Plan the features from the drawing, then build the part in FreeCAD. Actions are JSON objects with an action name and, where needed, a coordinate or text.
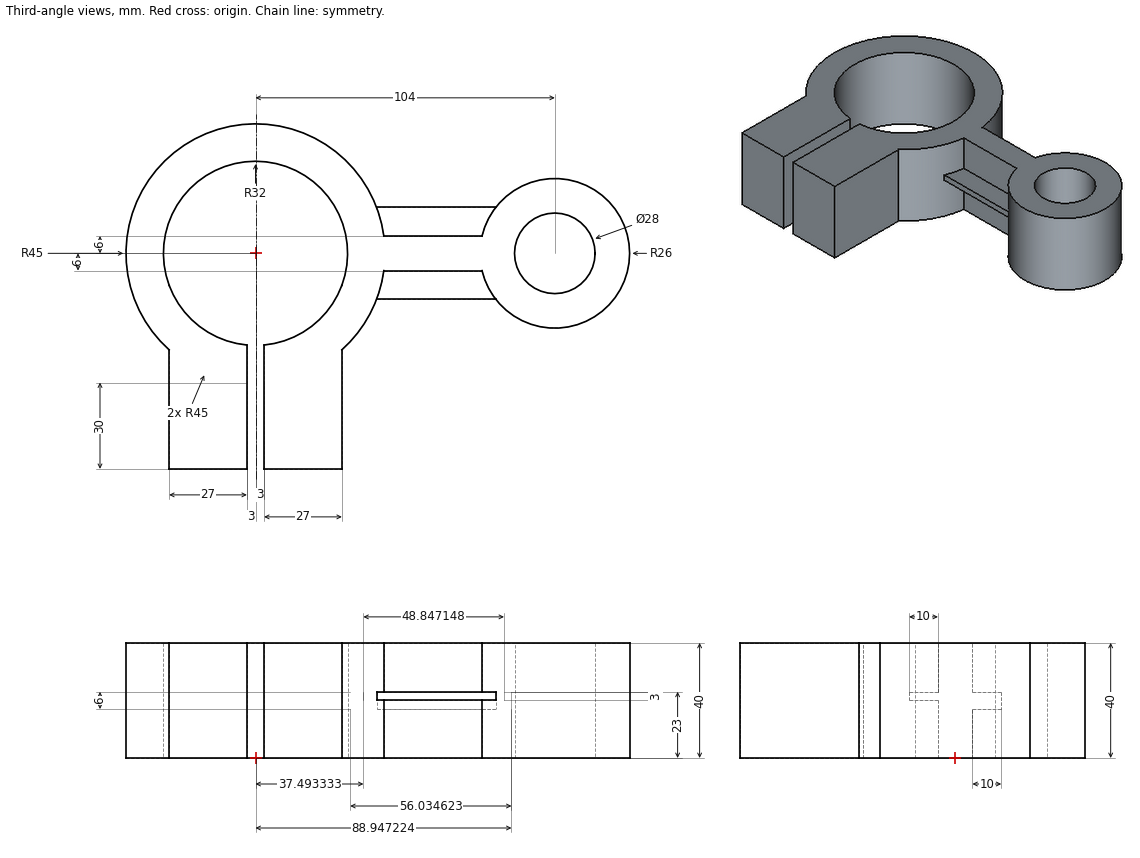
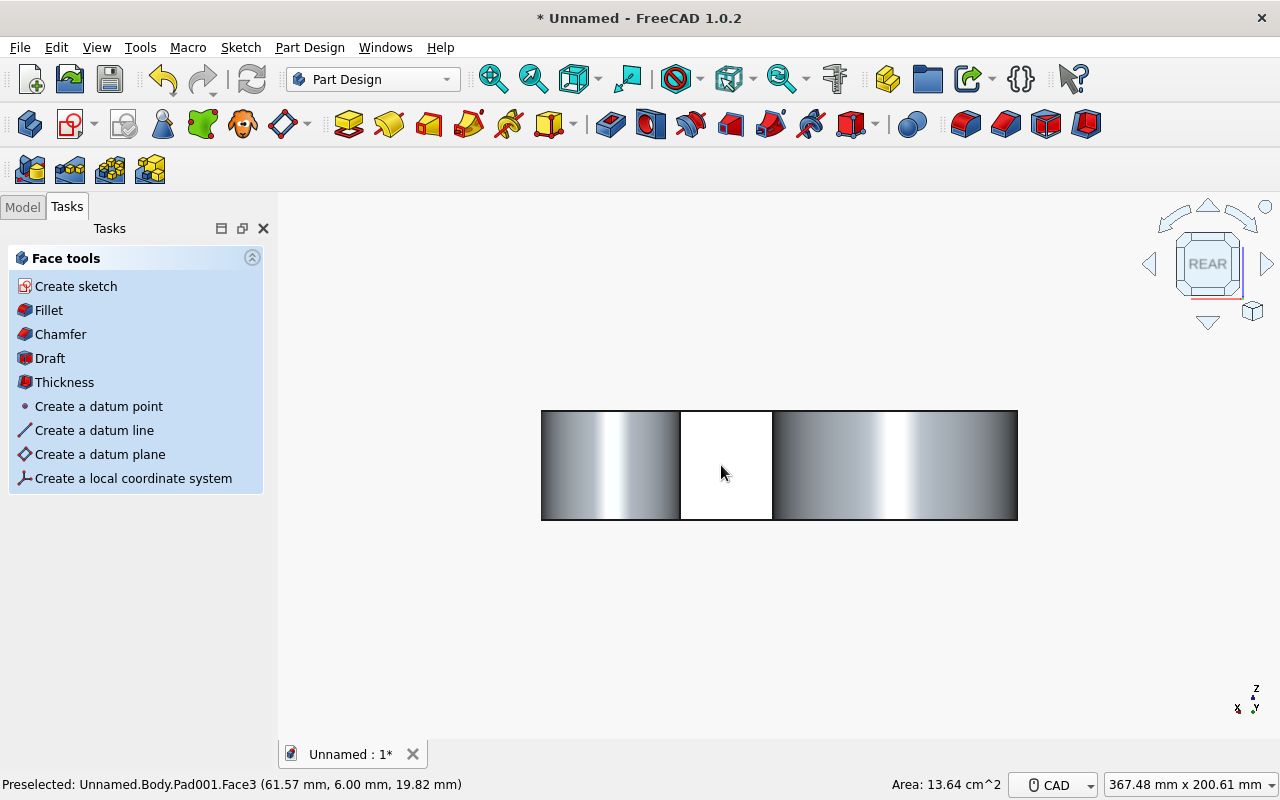
{"action": "left_click", "coordinate": [70, 124]}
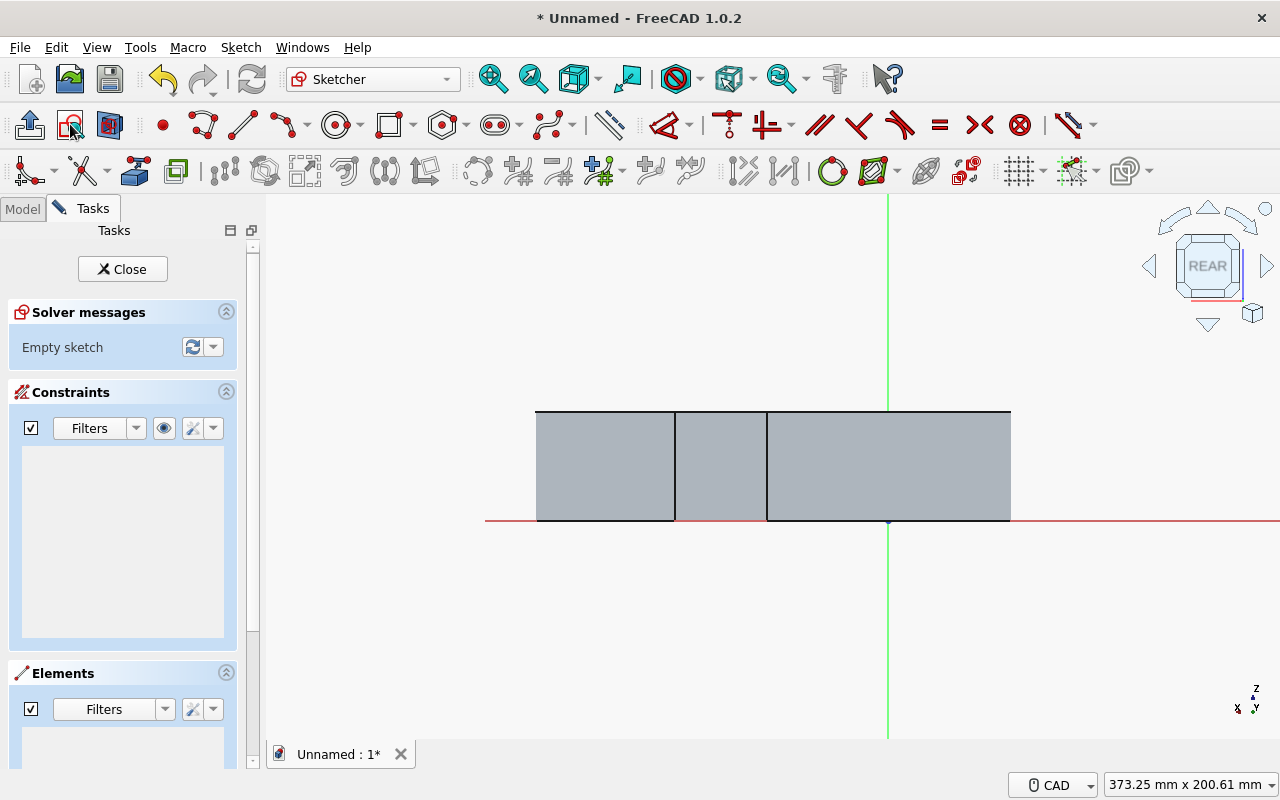
{"action": "scroll", "coordinate": [819, 508], "scroll_direction": "up", "scroll_amount": 4}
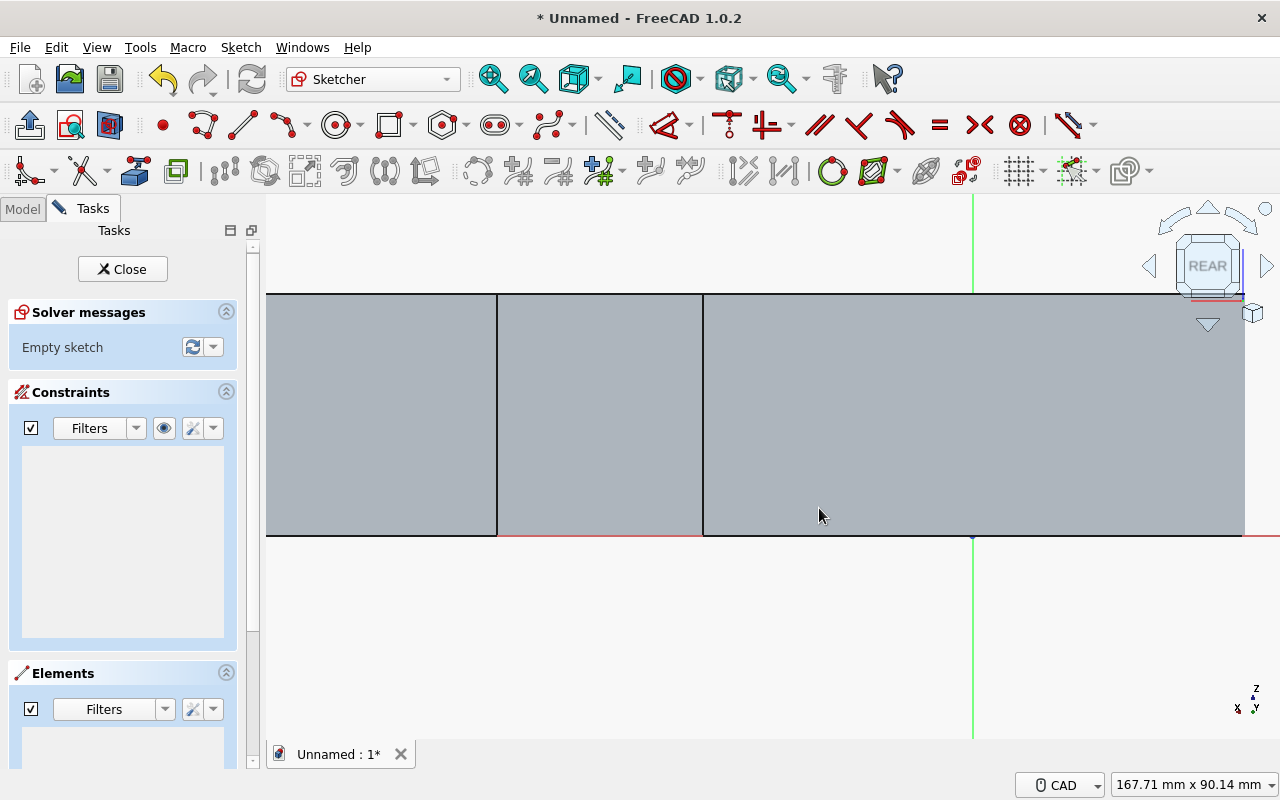
{"action": "key", "text": "g r"}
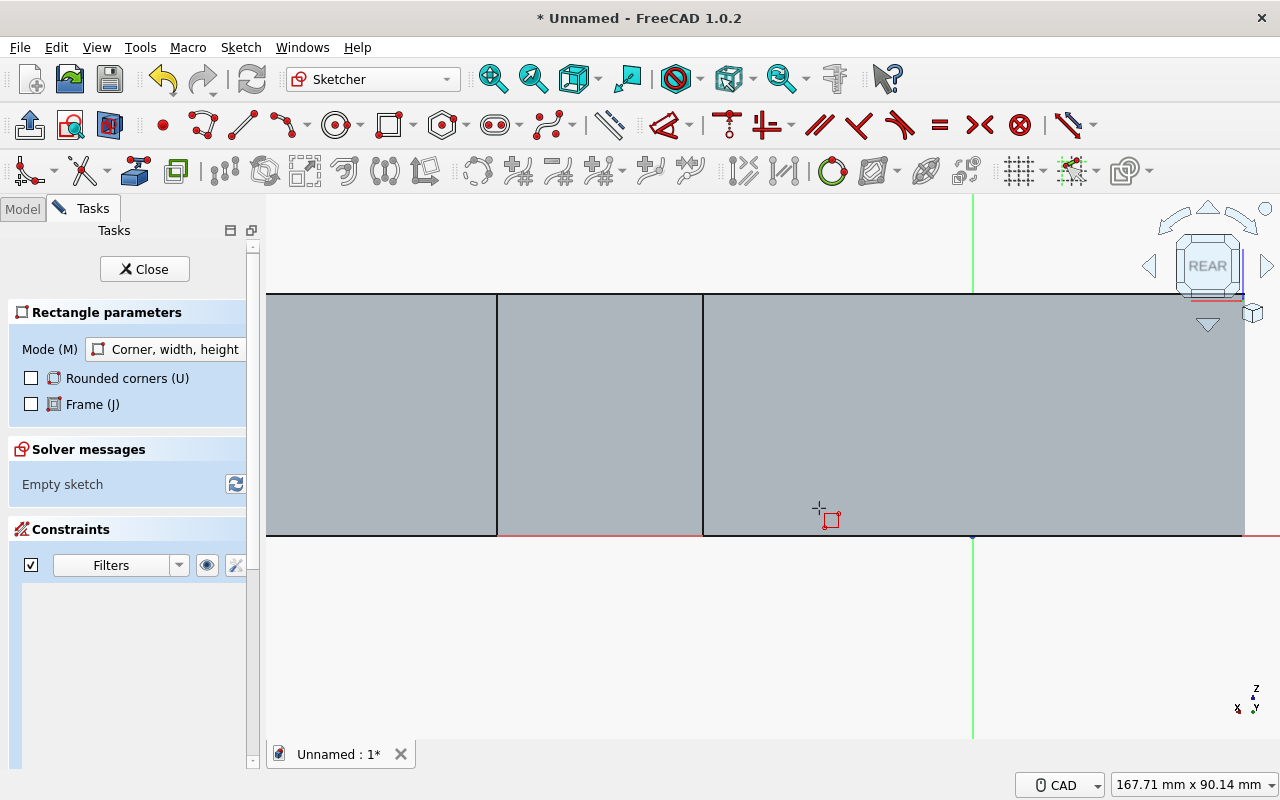
{"action": "left_click", "coordinate": [435, 397]}
{"action": "mouse_move", "coordinate": [774, 433]}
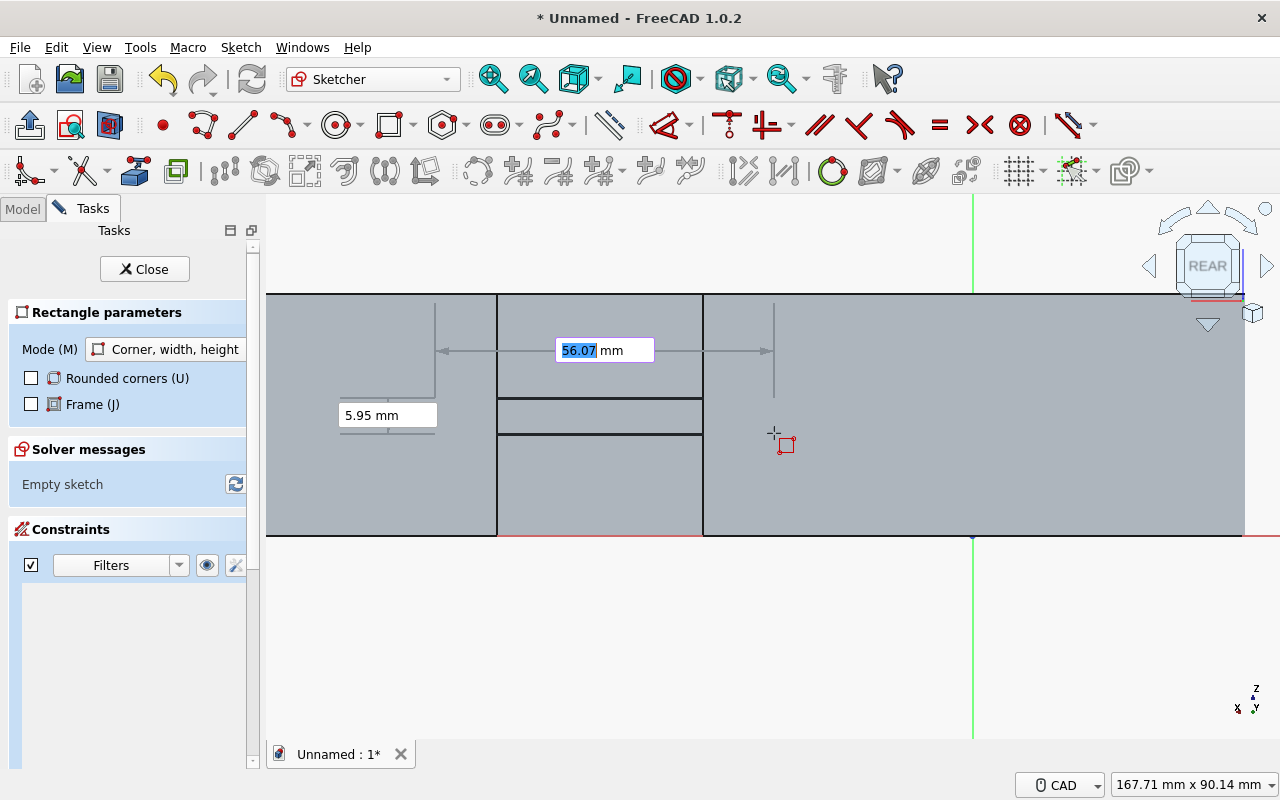
{"action": "type", "text": "56.034623"}
{"action": "key", "text": "Tab"}
{"action": "type", "text": "6"}
{"action": "key", "text": "Return"}
{"action": "key", "text": "Escape"}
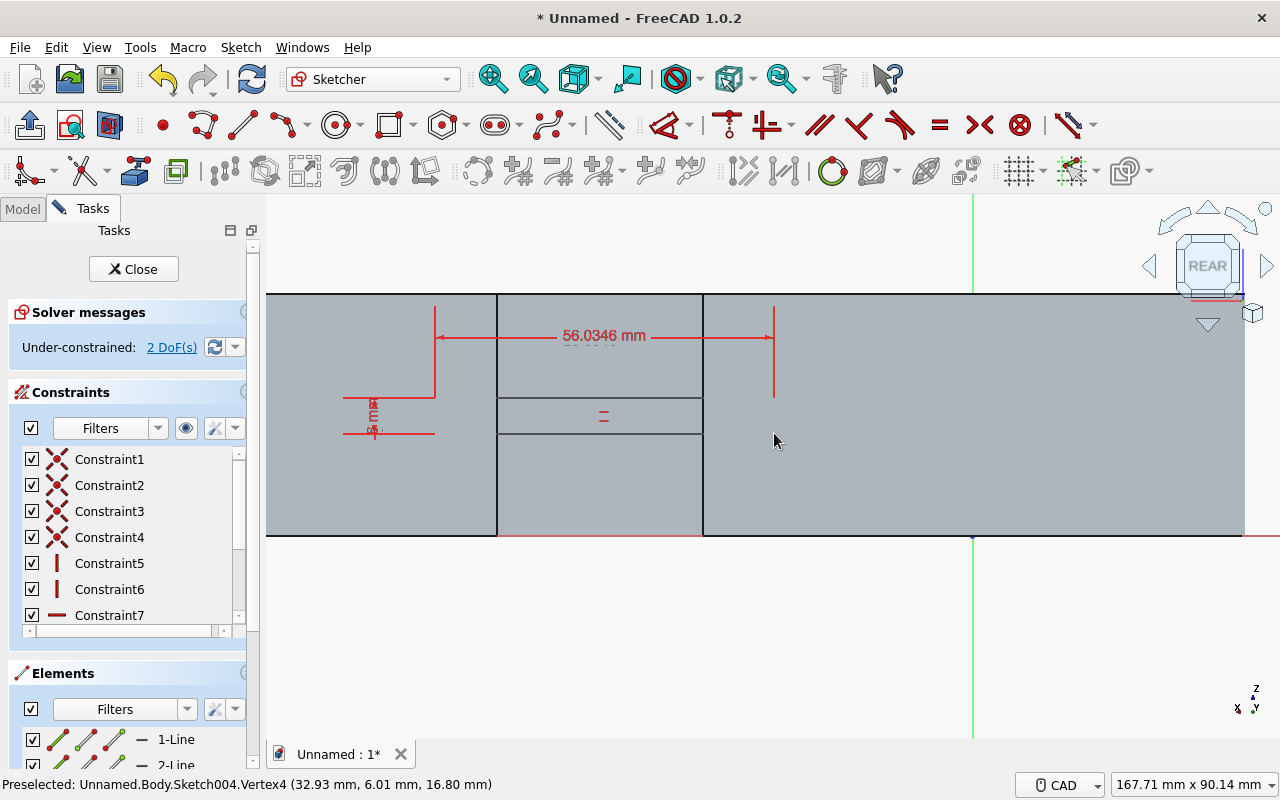
{"action": "key", "text": "d"}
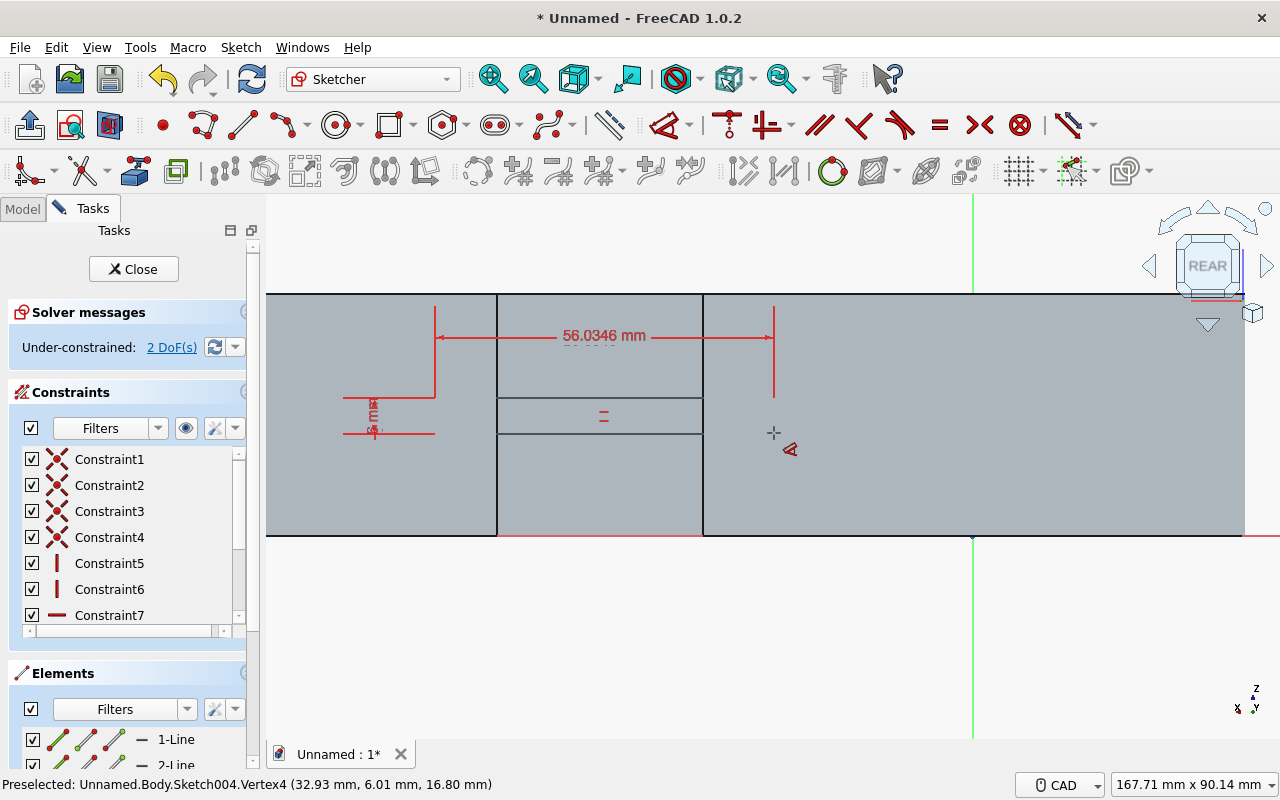
{"action": "left_click", "coordinate": [435, 398]}
{"action": "left_click", "coordinate": [401, 467]}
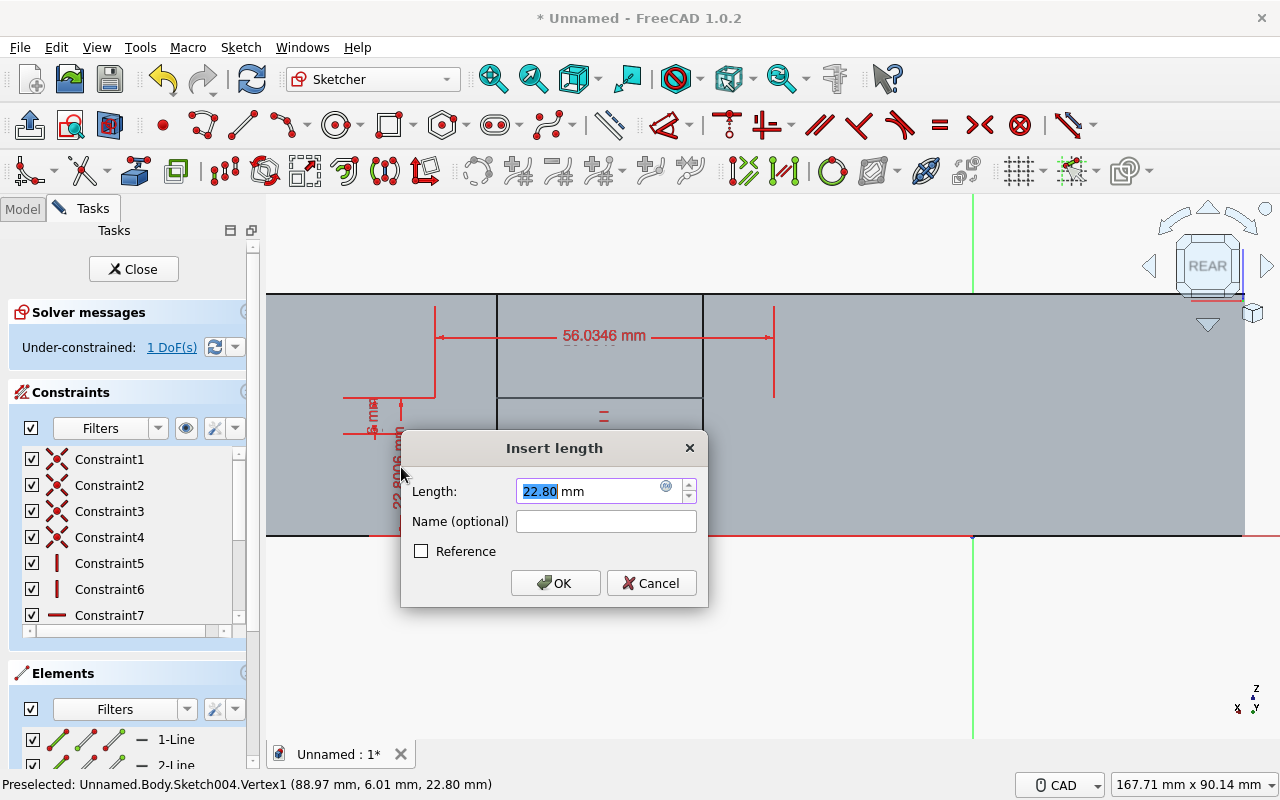
{"action": "type", "text": "23"}
{"action": "key", "text": "Return"}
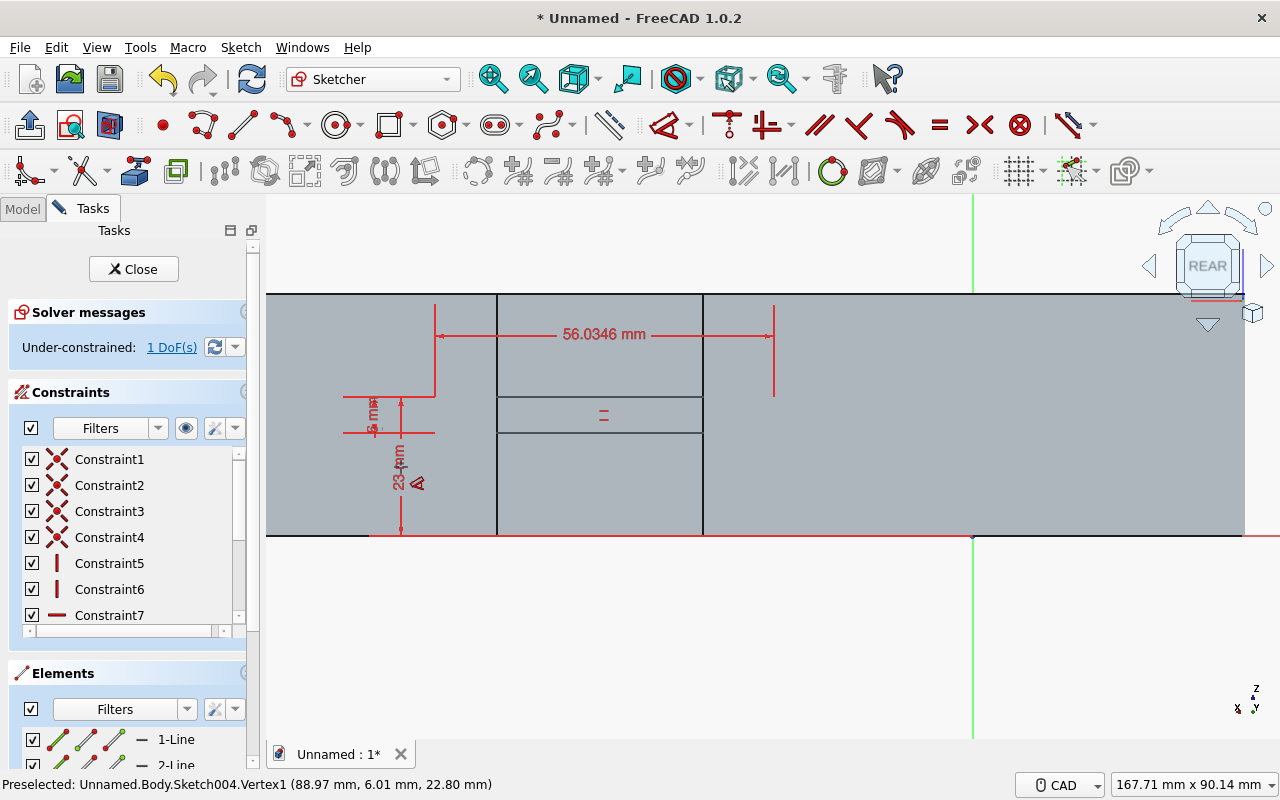
{"action": "left_click", "coordinate": [435, 397]}
{"action": "left_click", "coordinate": [704, 570]}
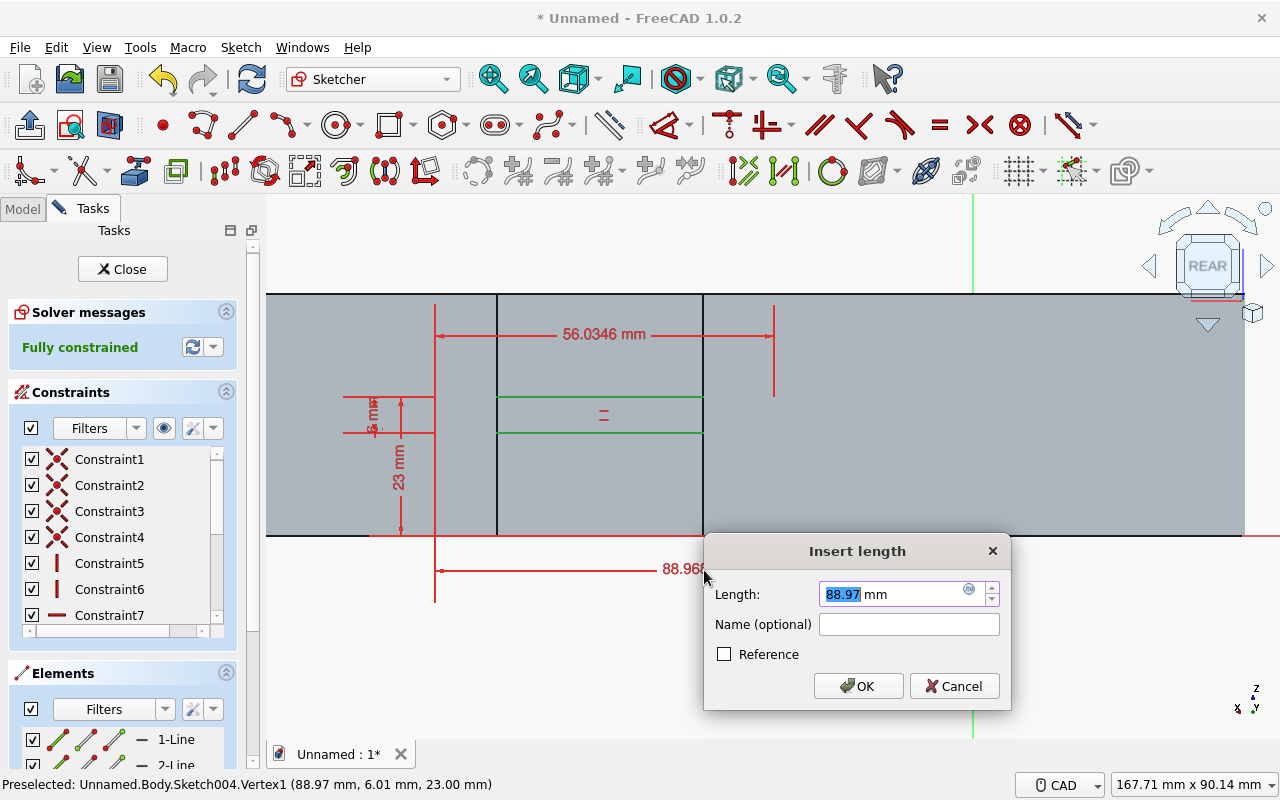
{"action": "type", "text": "88.947224"}
{"action": "key", "text": "Return"}
{"action": "key", "text": "Escape"}